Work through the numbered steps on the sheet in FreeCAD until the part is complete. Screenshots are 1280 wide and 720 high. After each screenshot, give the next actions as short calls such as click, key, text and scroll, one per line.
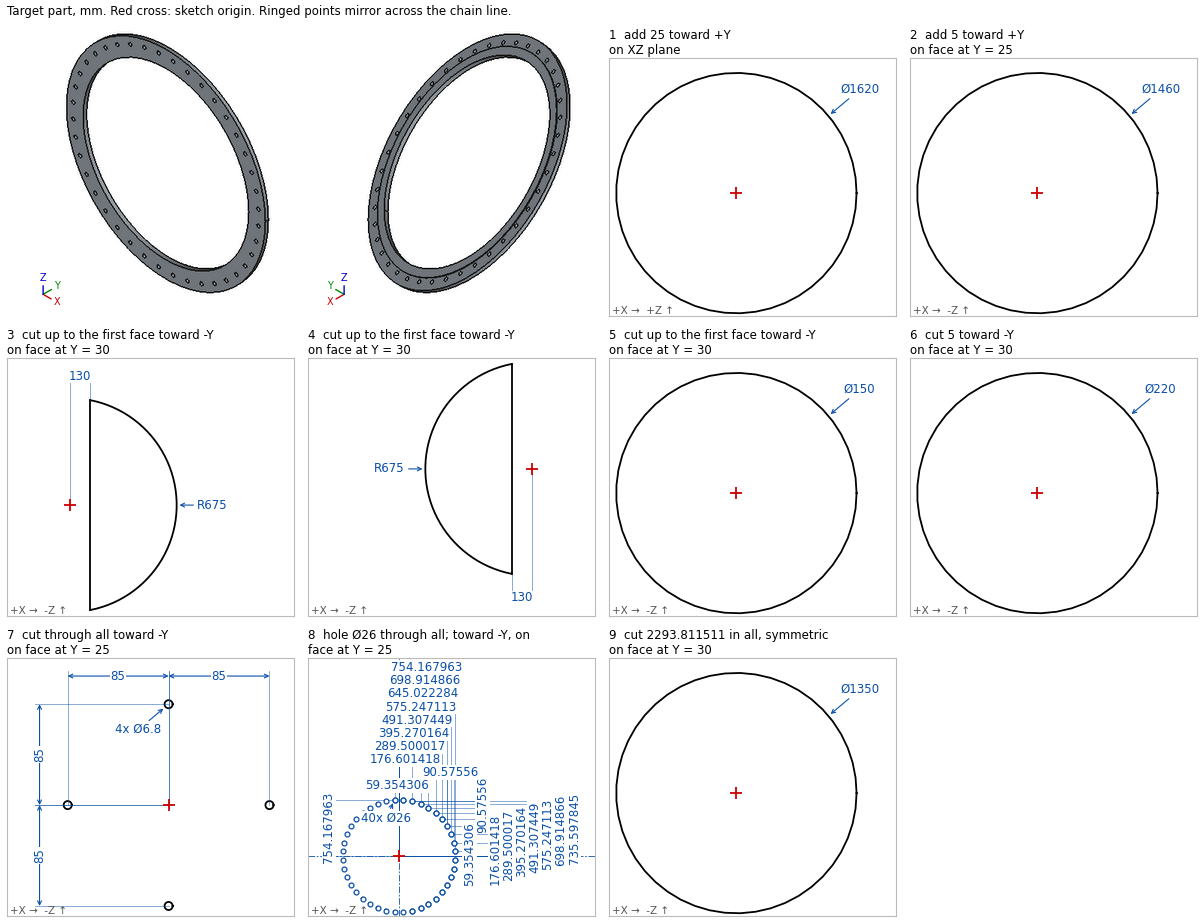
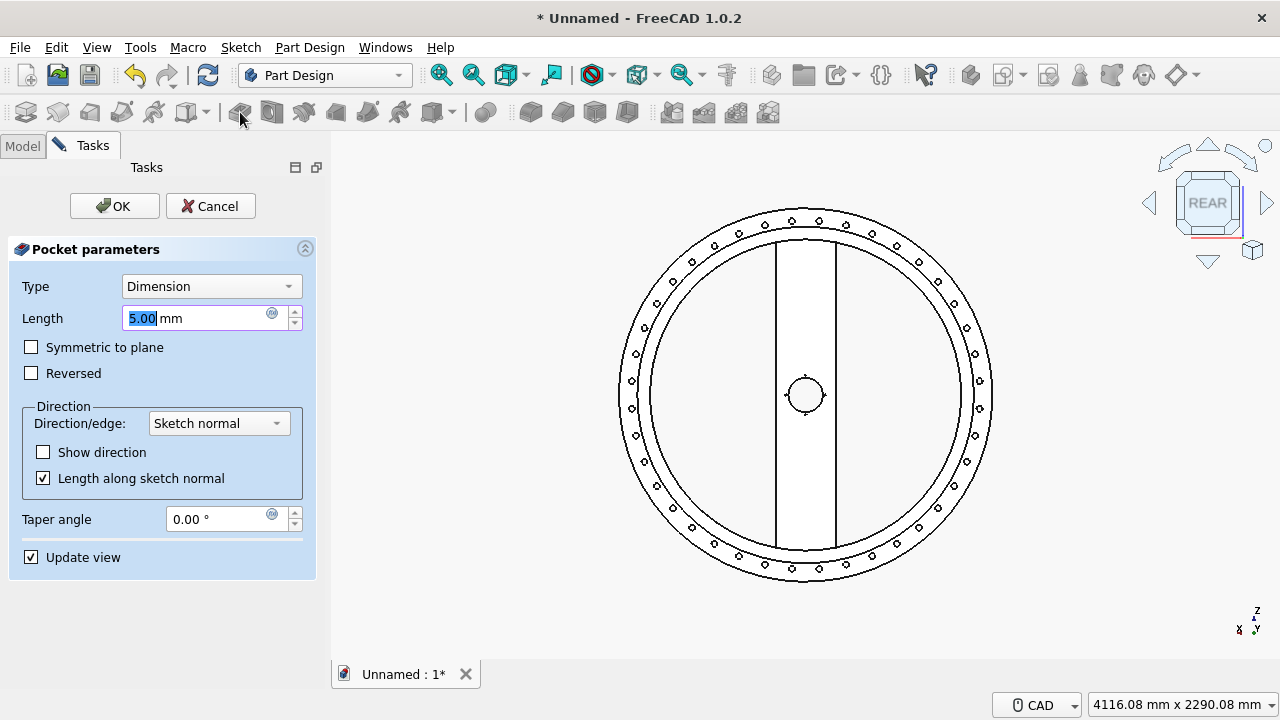
text(2293.811511)
key(Tab)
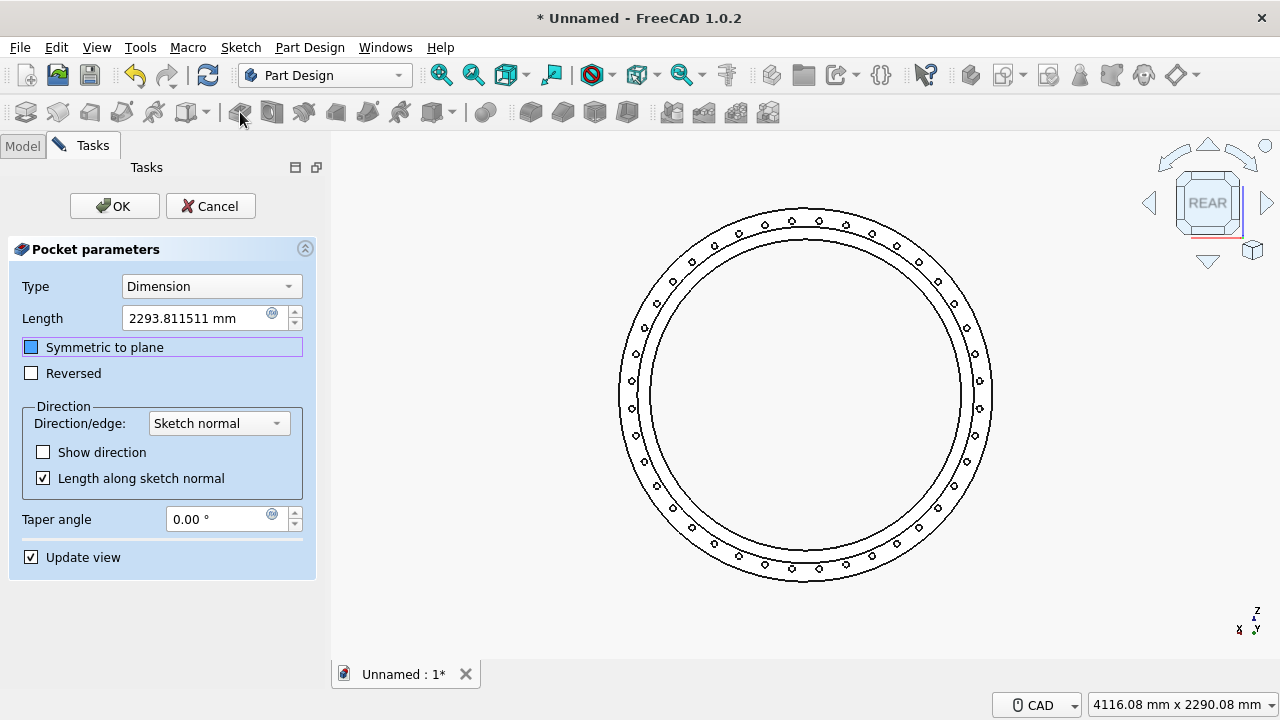
click(30, 347)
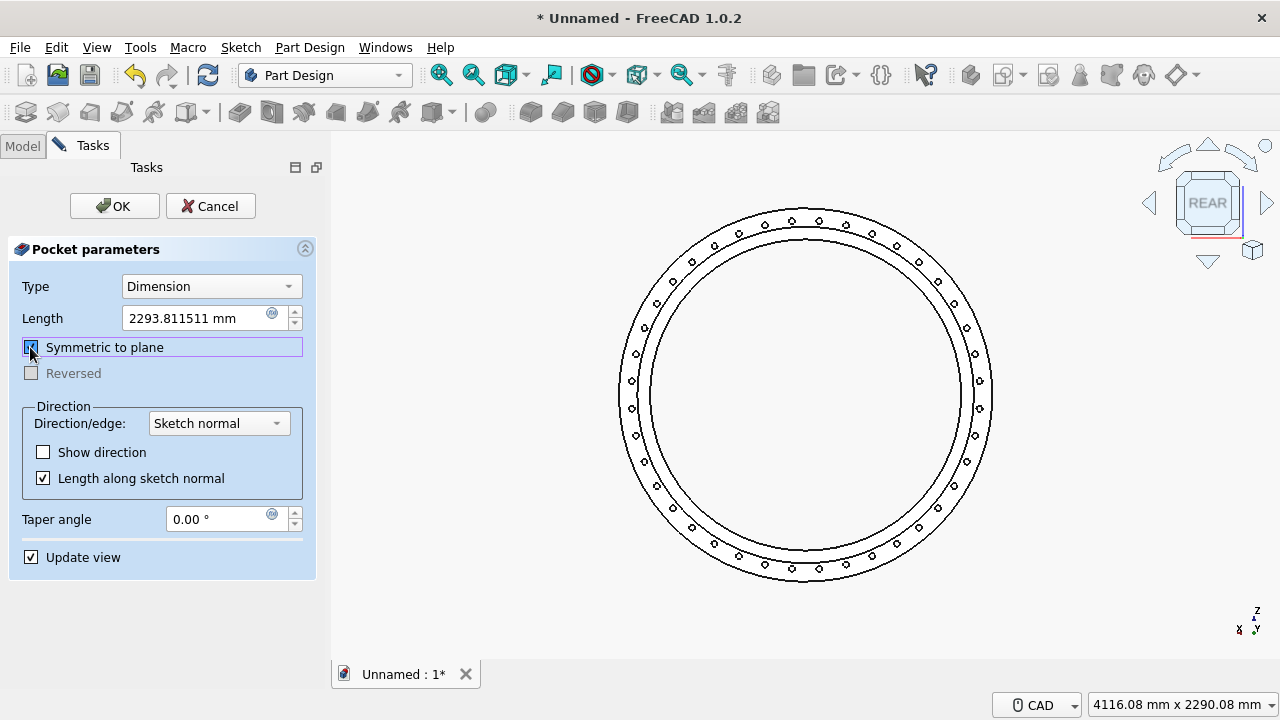
click(115, 206)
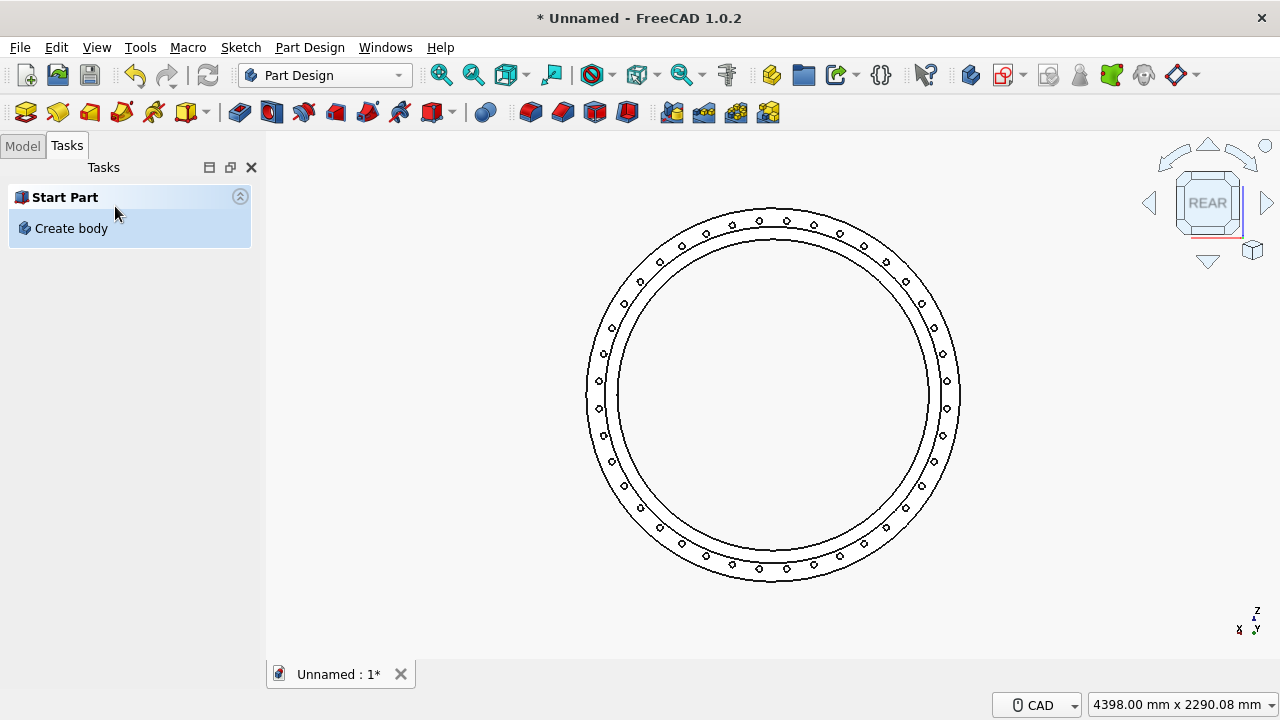
key(0)